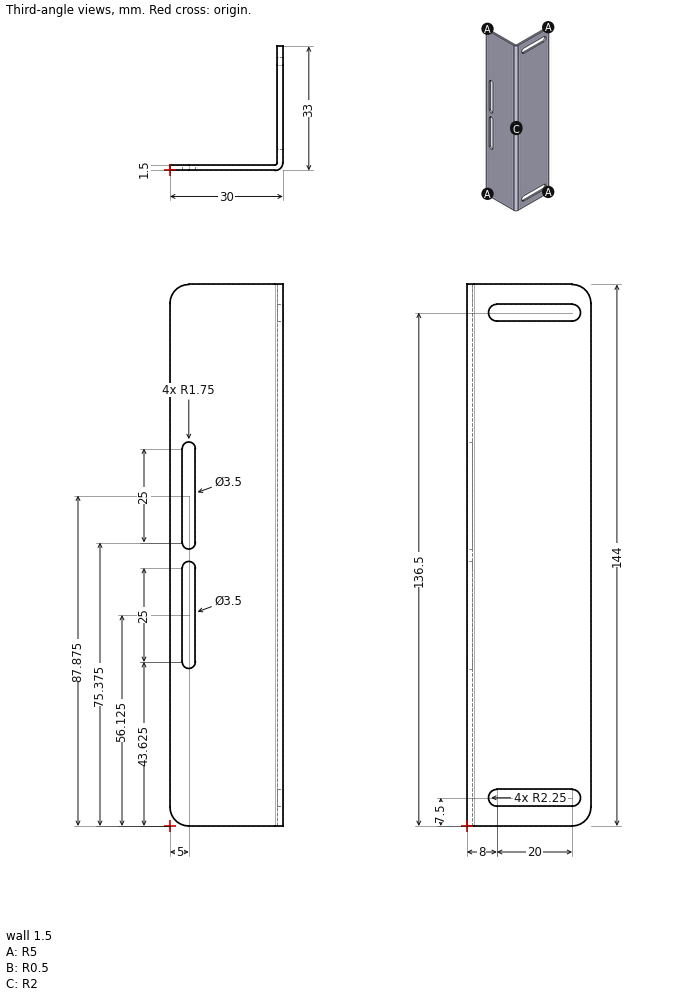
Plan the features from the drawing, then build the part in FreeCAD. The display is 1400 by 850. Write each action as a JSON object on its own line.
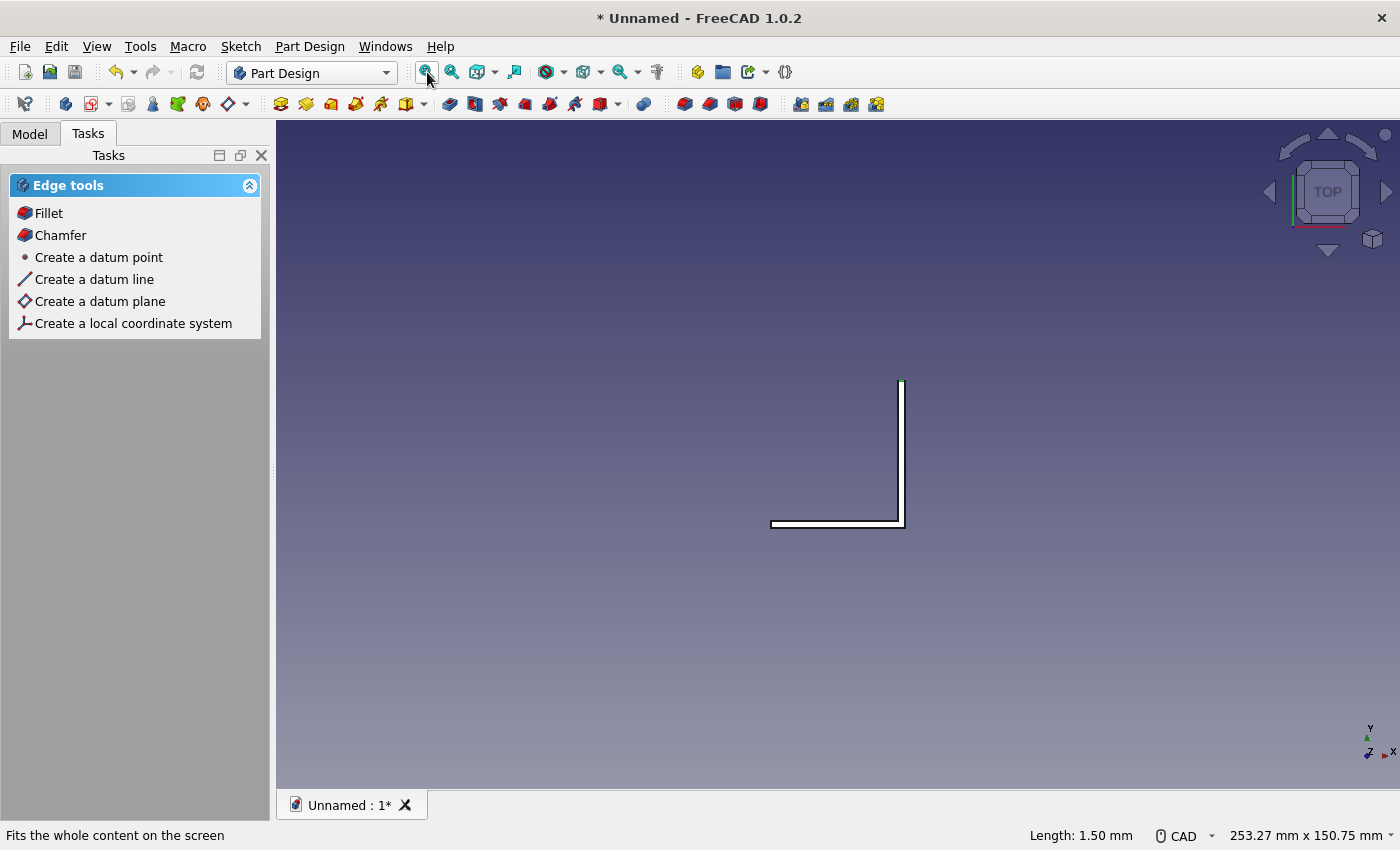
{"action": "key", "text": "1"}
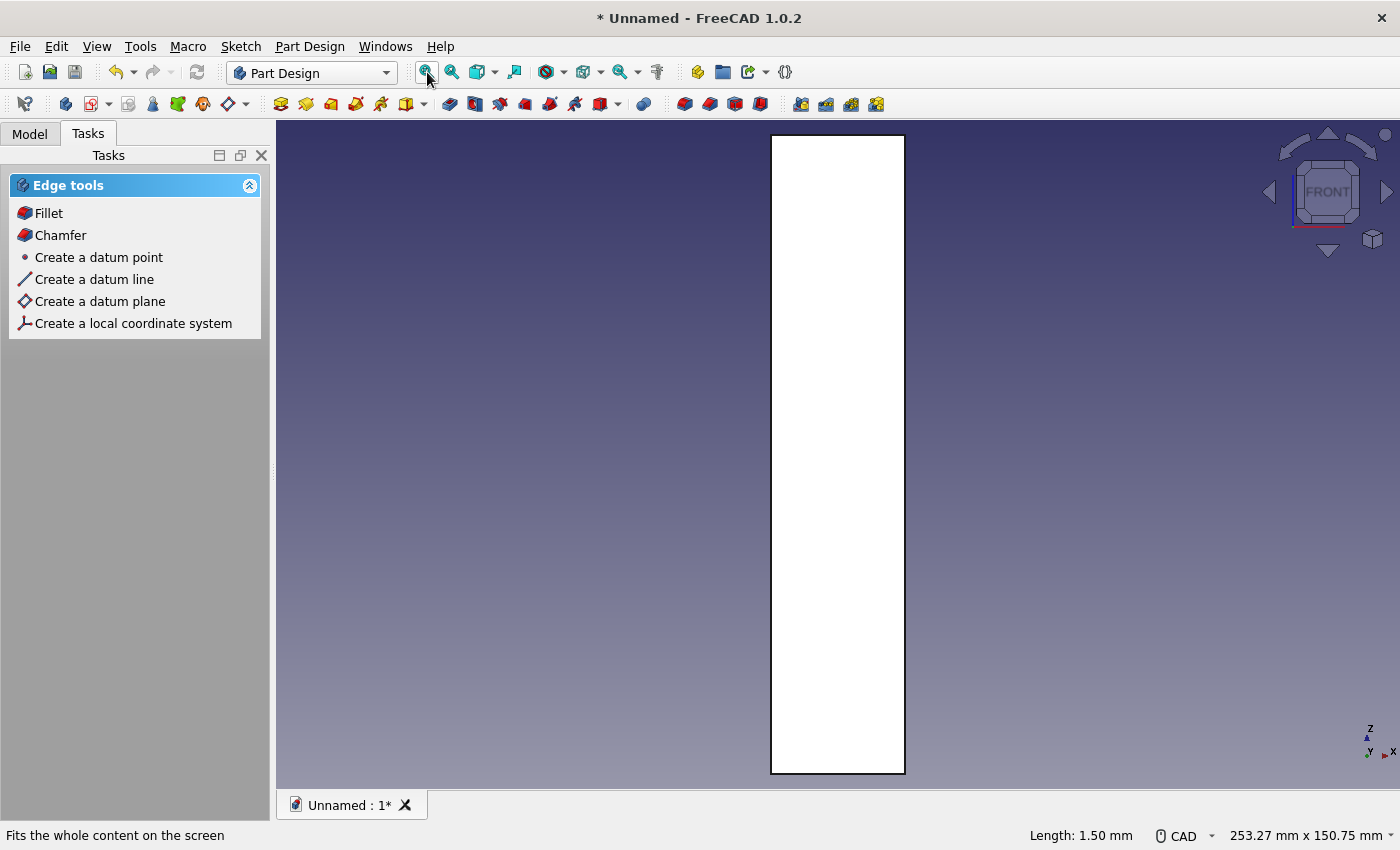
{"action": "key", "text": "3"}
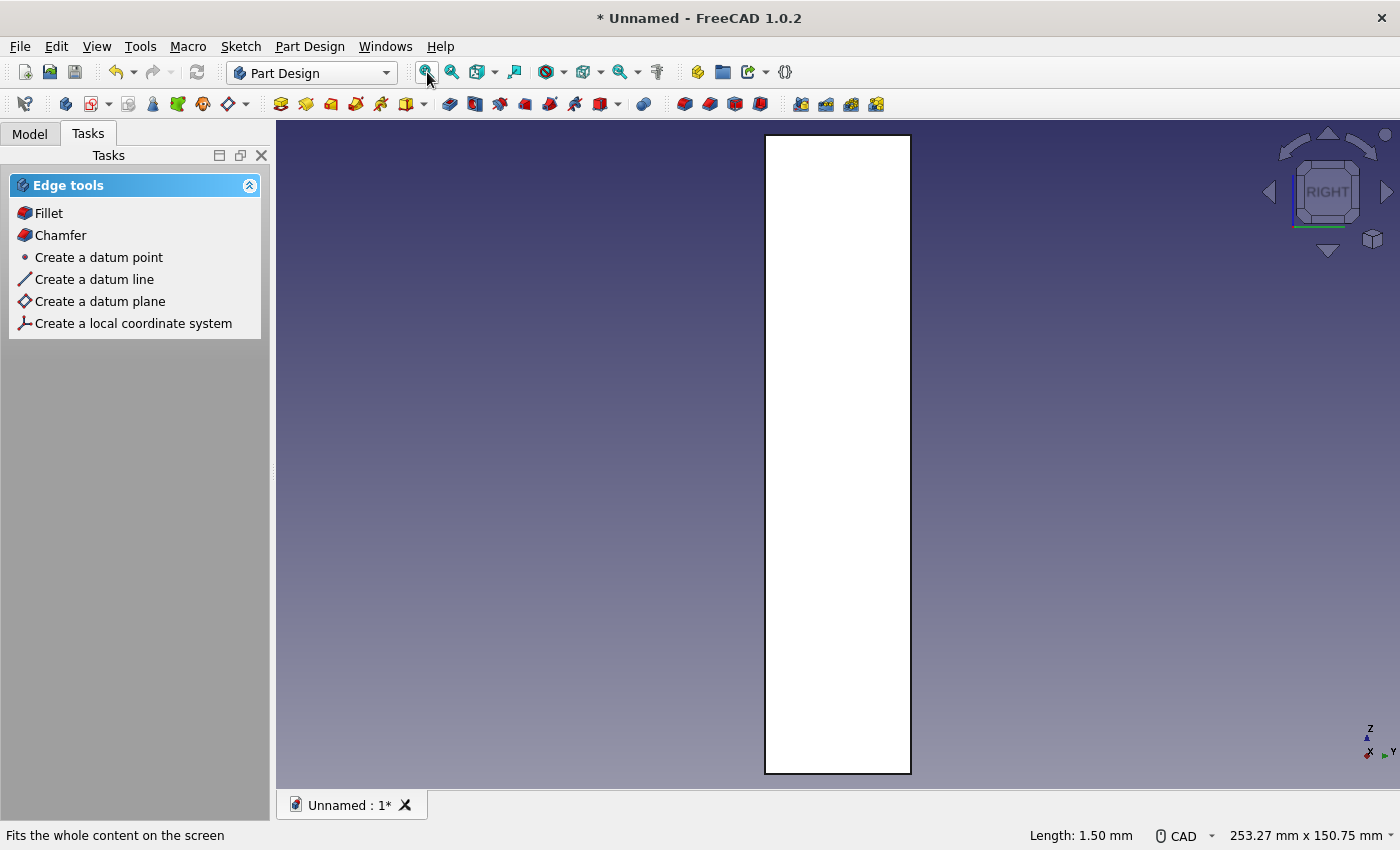
{"action": "key", "text": "5"}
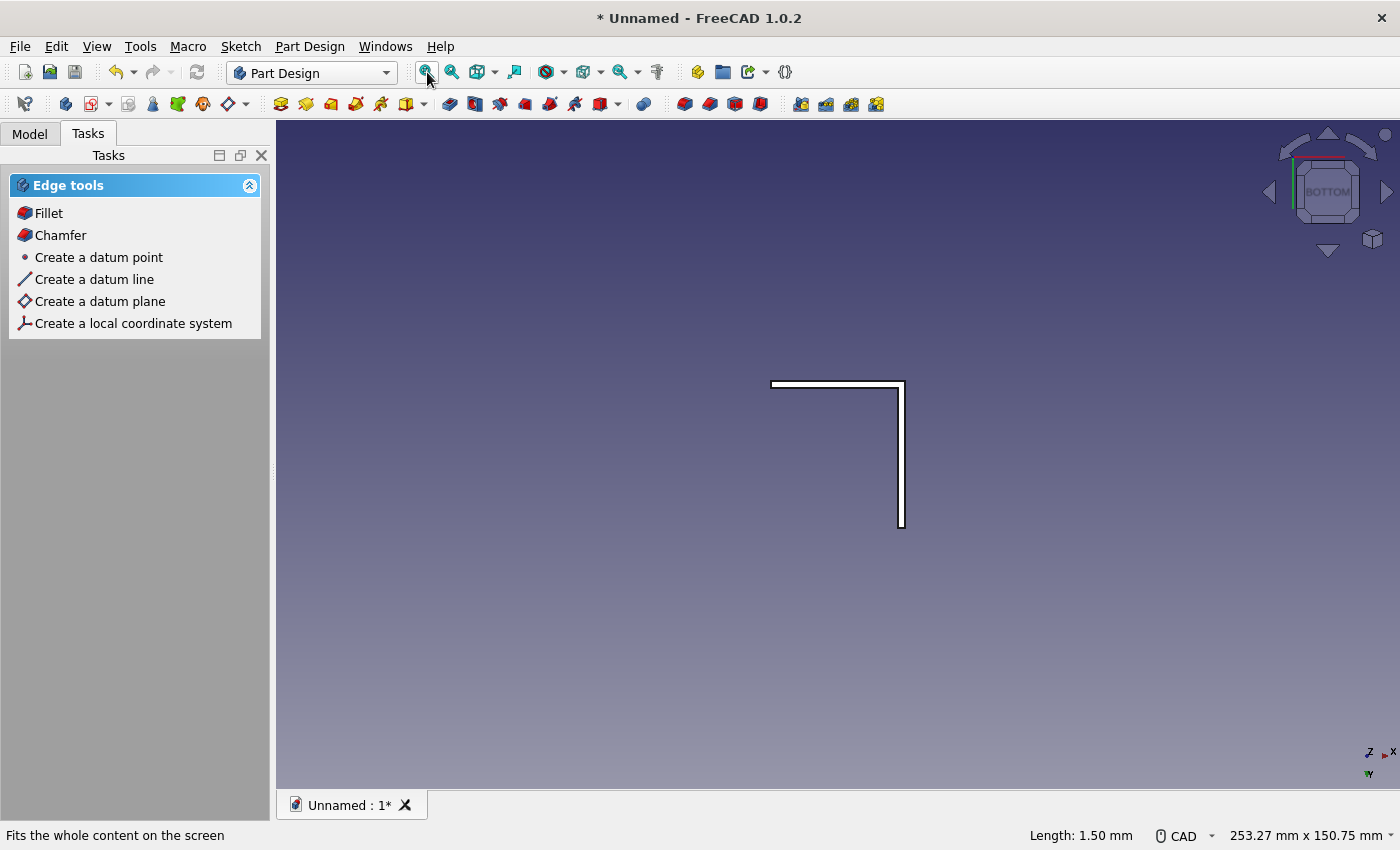
{"action": "left_click", "coordinate": [427, 72]}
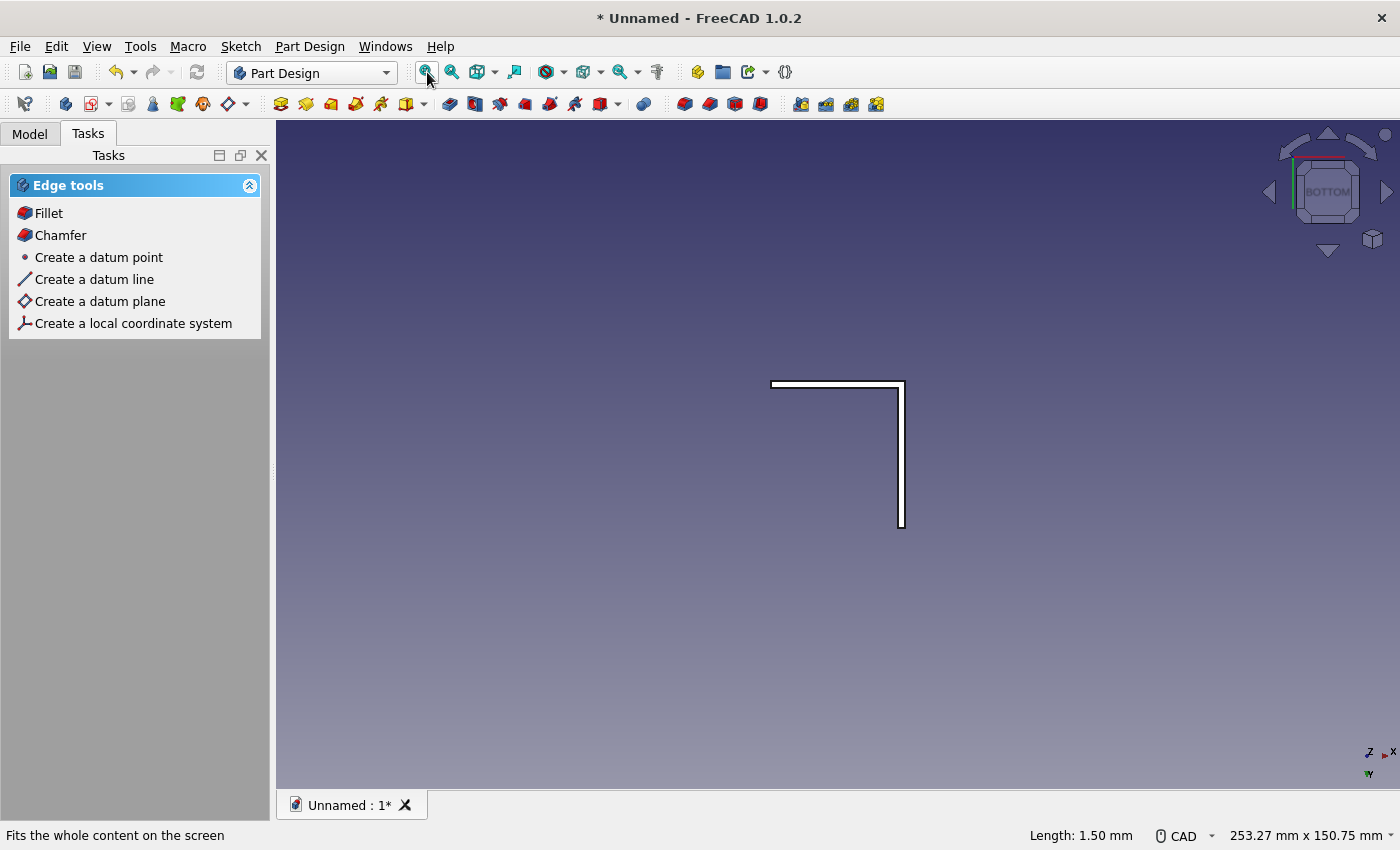
{"action": "scroll", "coordinate": [771, 384], "scroll_direction": "up", "scroll_amount": 9}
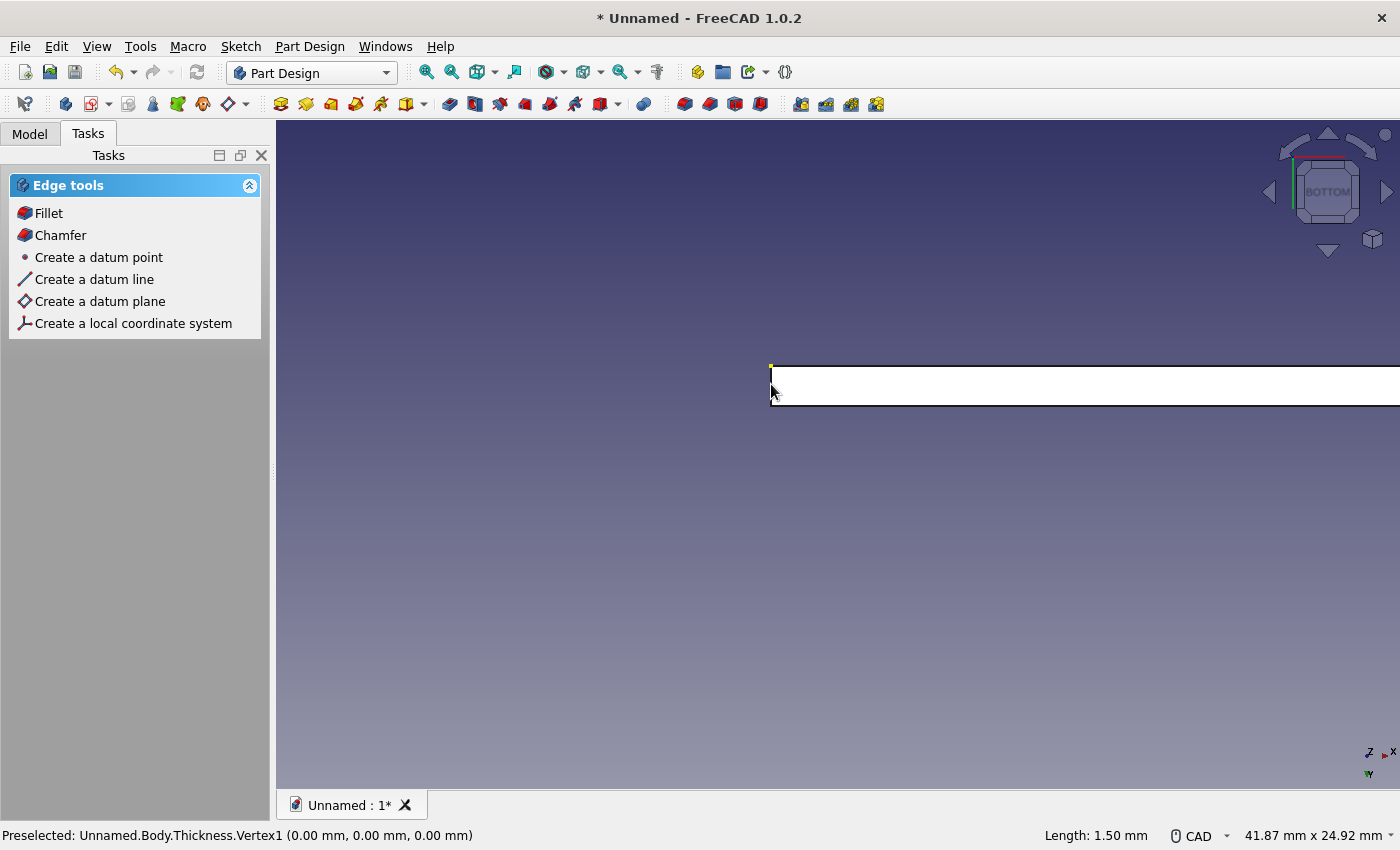
{"action": "left_click", "coordinate": [771, 385], "text": "ctrl"}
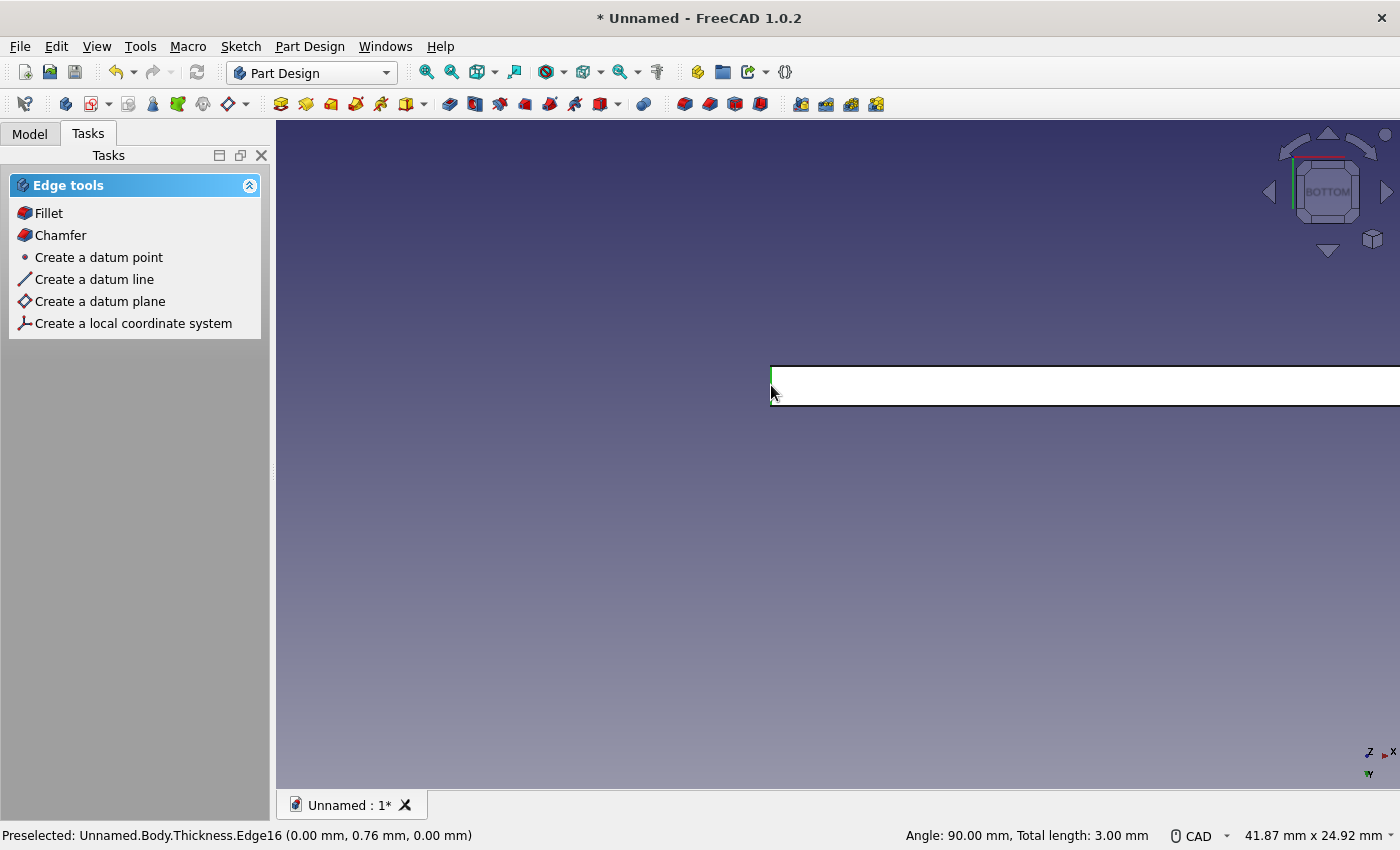
{"action": "left_click", "coordinate": [427, 72]}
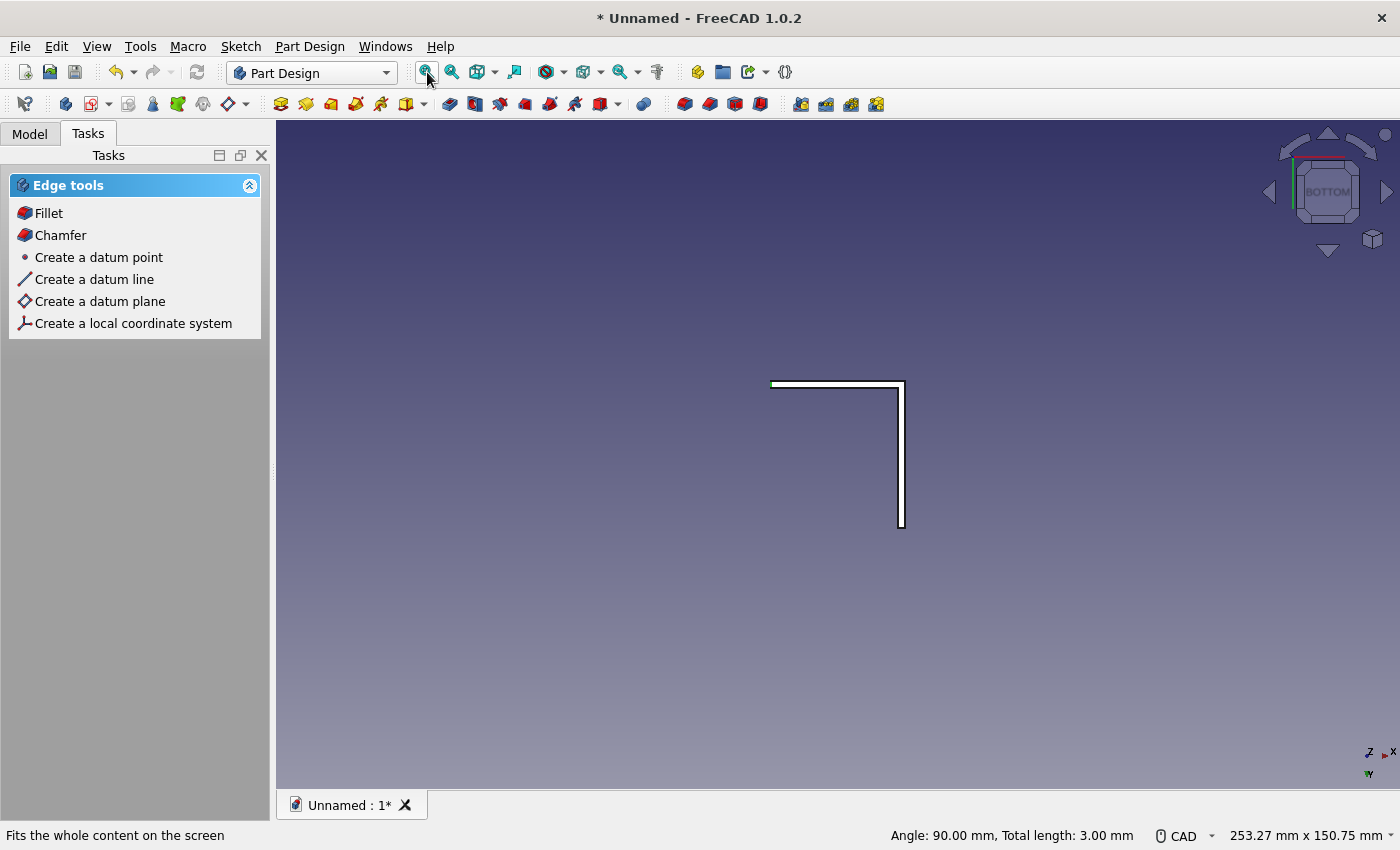
{"action": "key", "text": "4"}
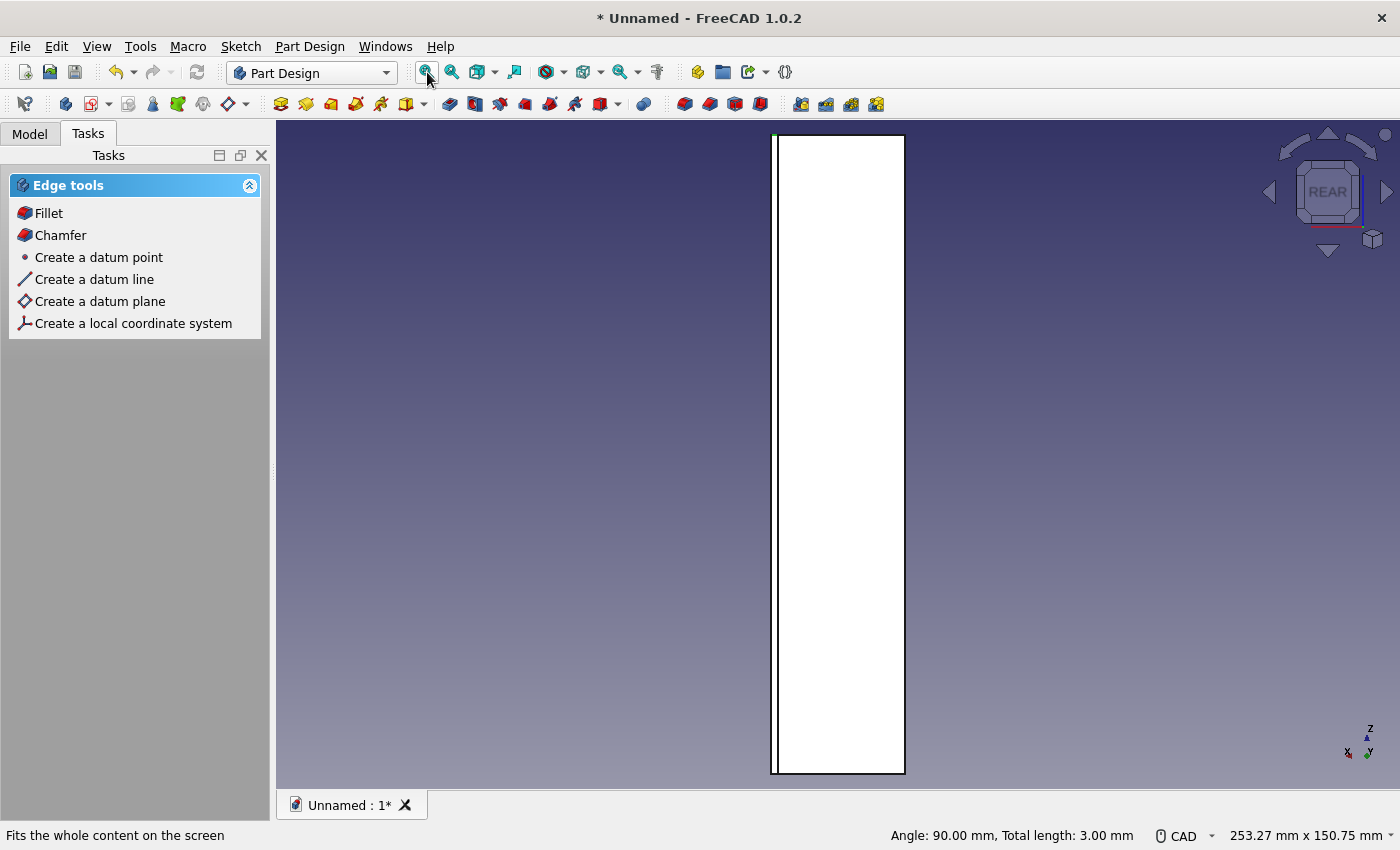
{"action": "key", "text": "6"}